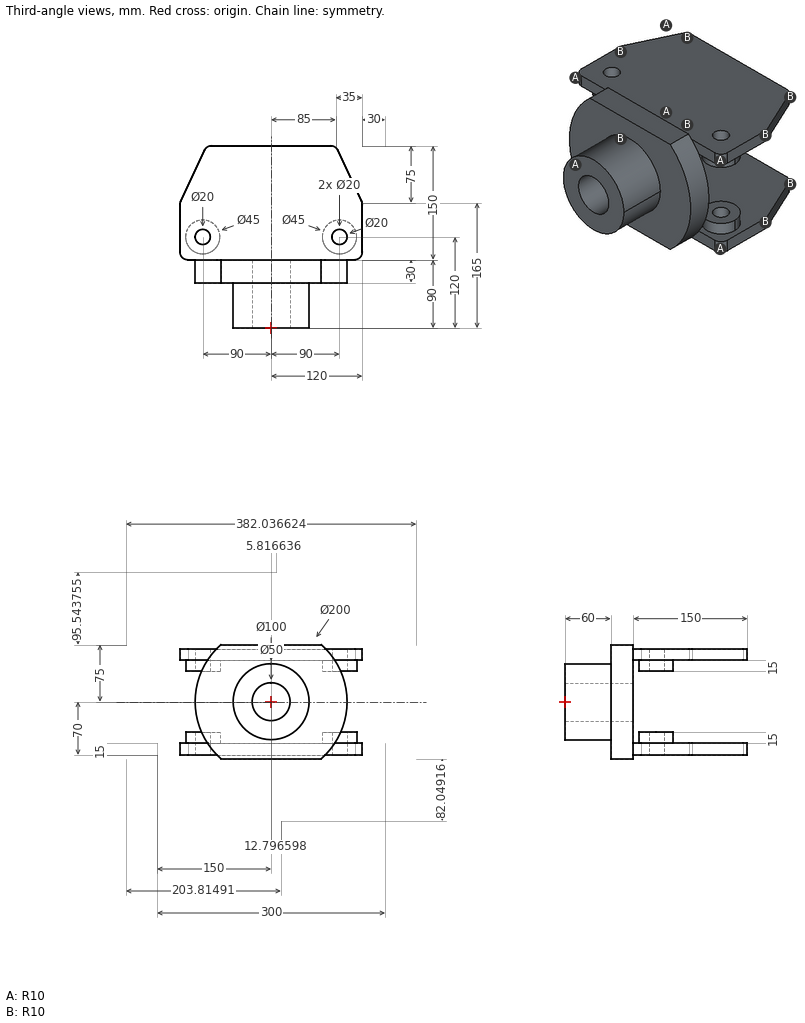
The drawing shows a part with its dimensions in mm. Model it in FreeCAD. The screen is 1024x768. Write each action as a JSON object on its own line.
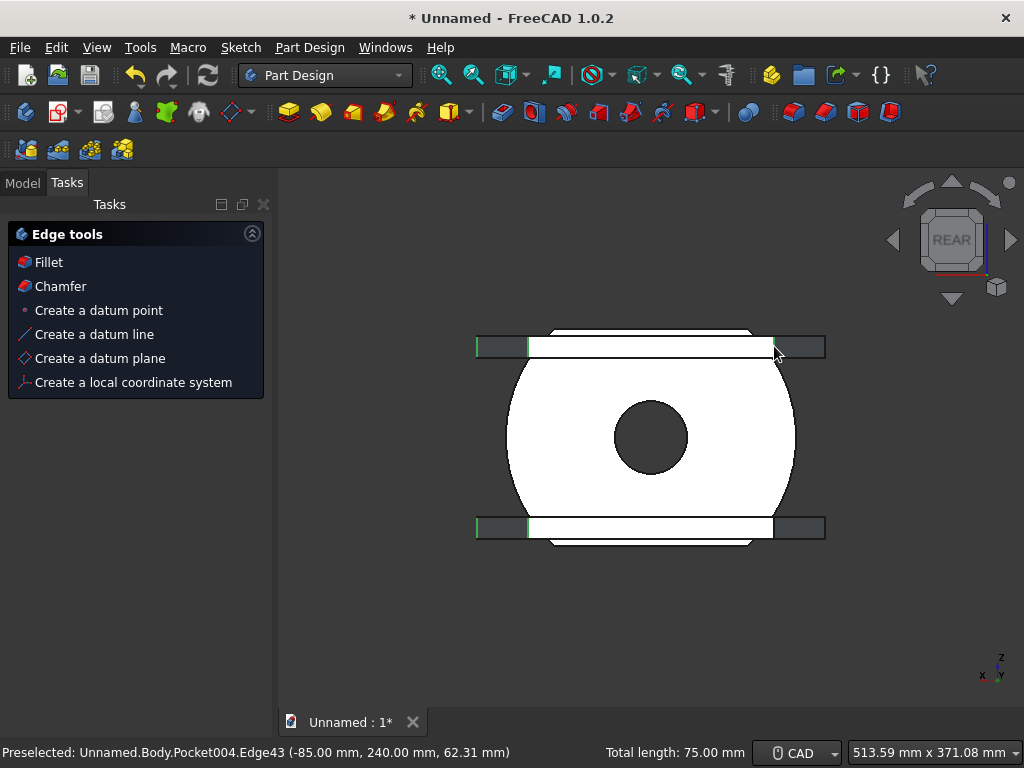
{"action": "left_click", "coordinate": [774, 527], "text": "ctrl"}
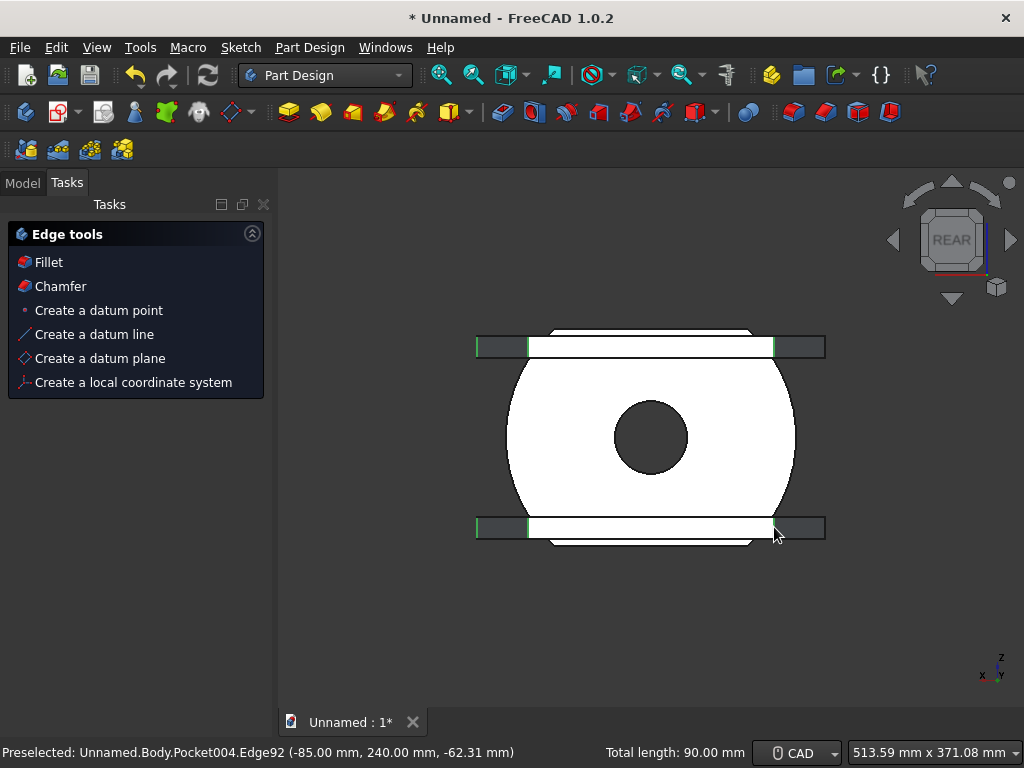
{"action": "scroll", "coordinate": [825, 527], "scroll_direction": "up", "scroll_amount": 4}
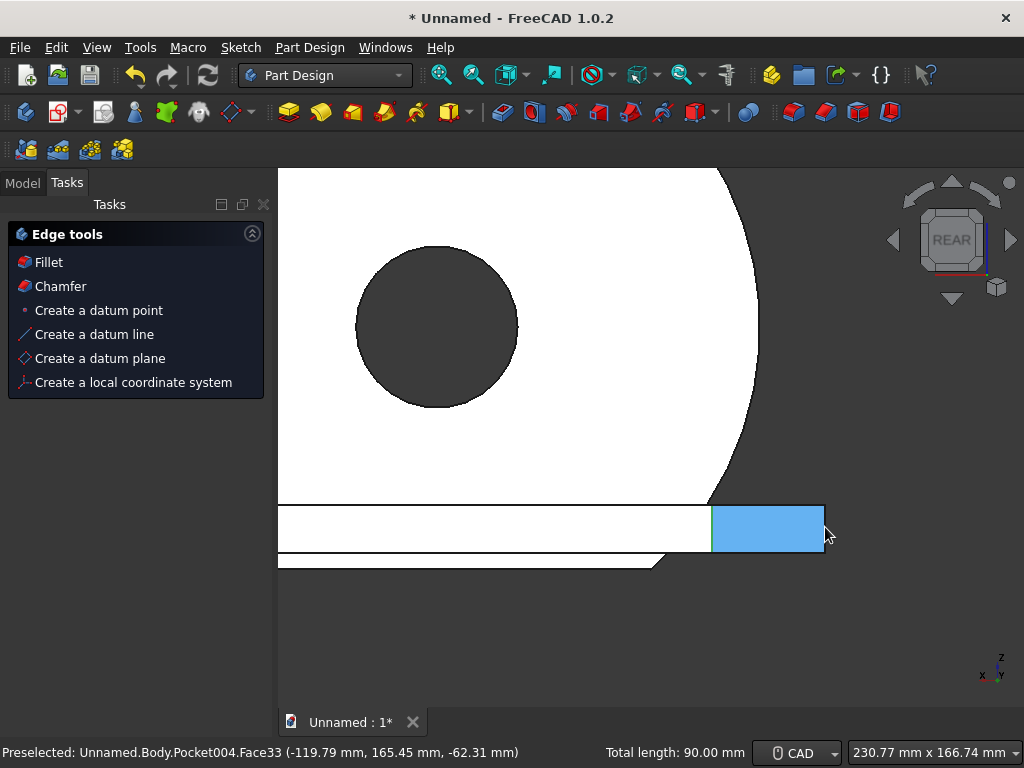
{"action": "left_click", "coordinate": [442, 76]}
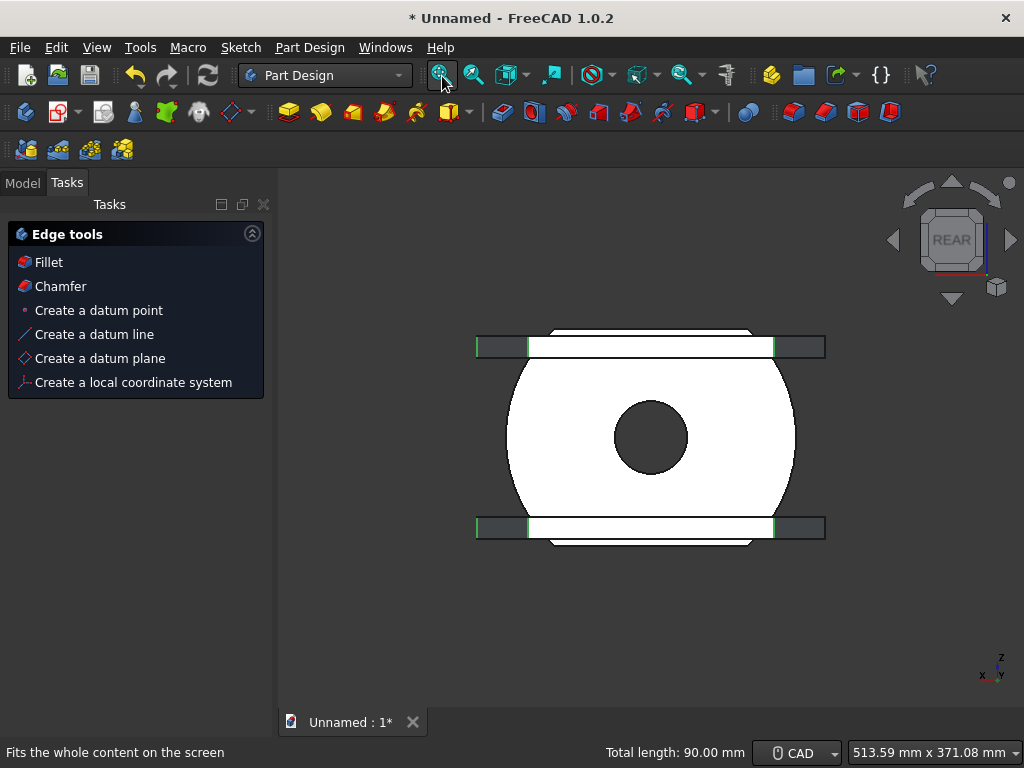
{"action": "key", "text": "6"}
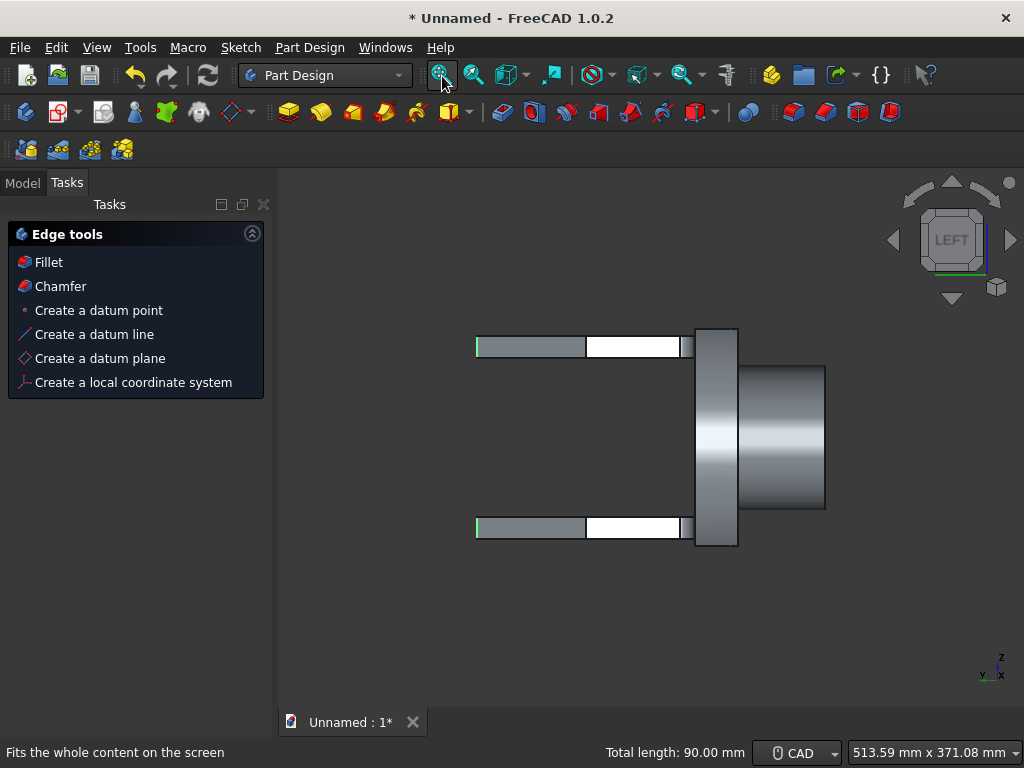
{"action": "left_click", "coordinate": [586, 527], "text": "ctrl"}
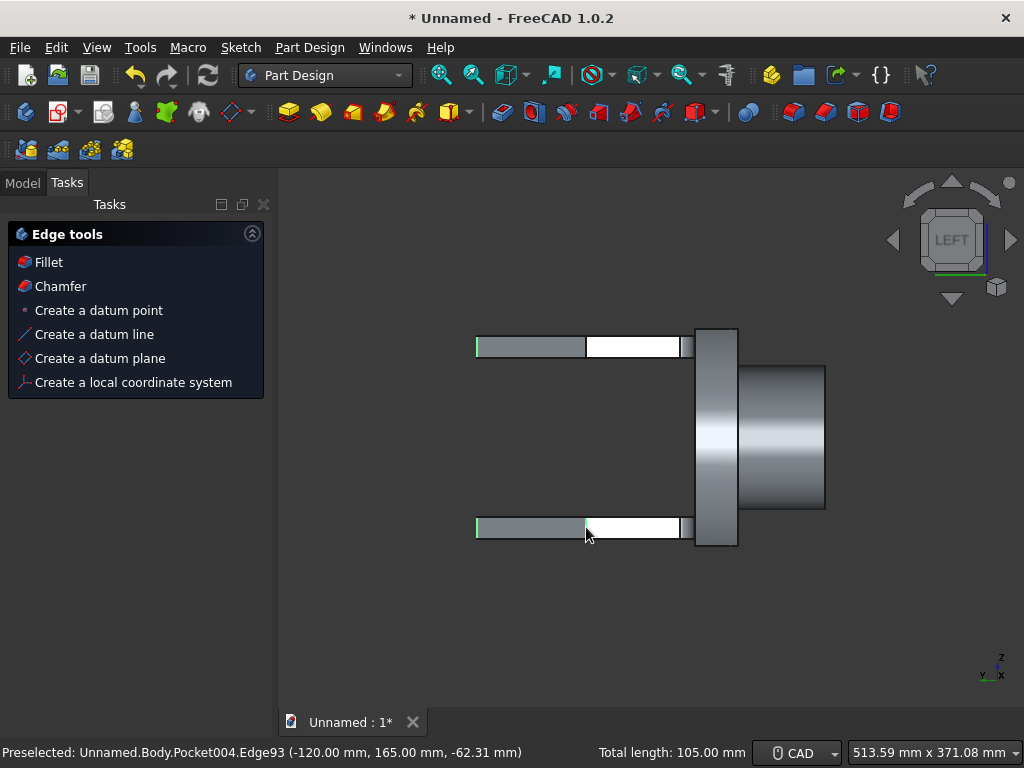
{"action": "left_click", "coordinate": [586, 346], "text": "ctrl"}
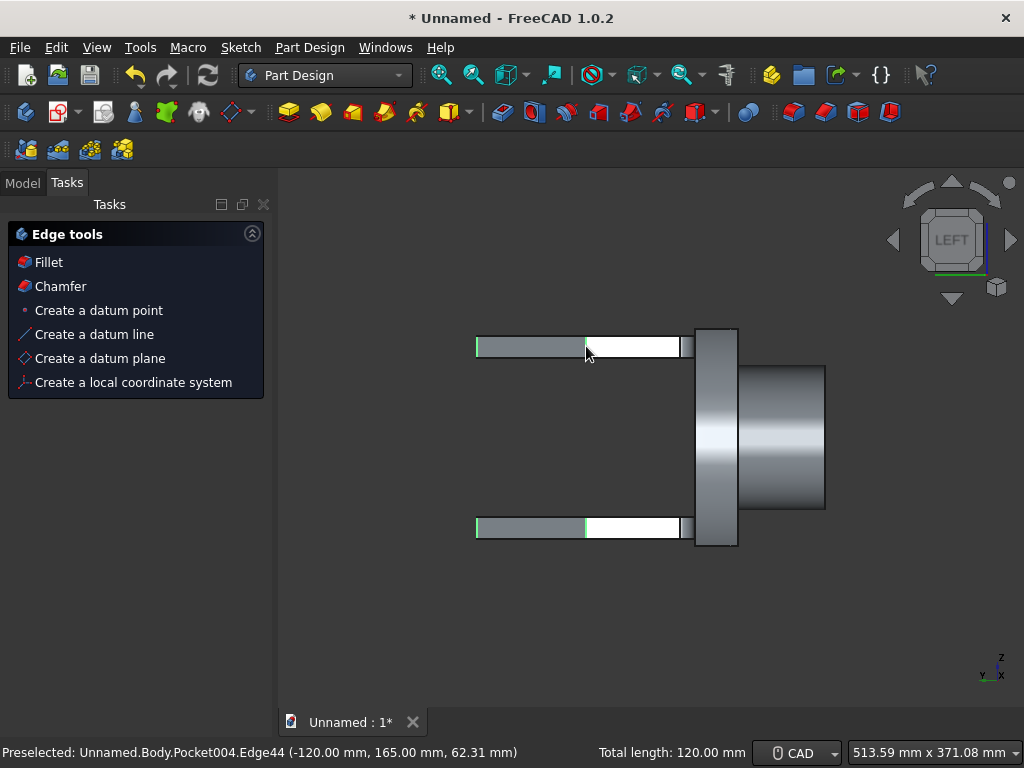
{"action": "left_click", "coordinate": [794, 112]}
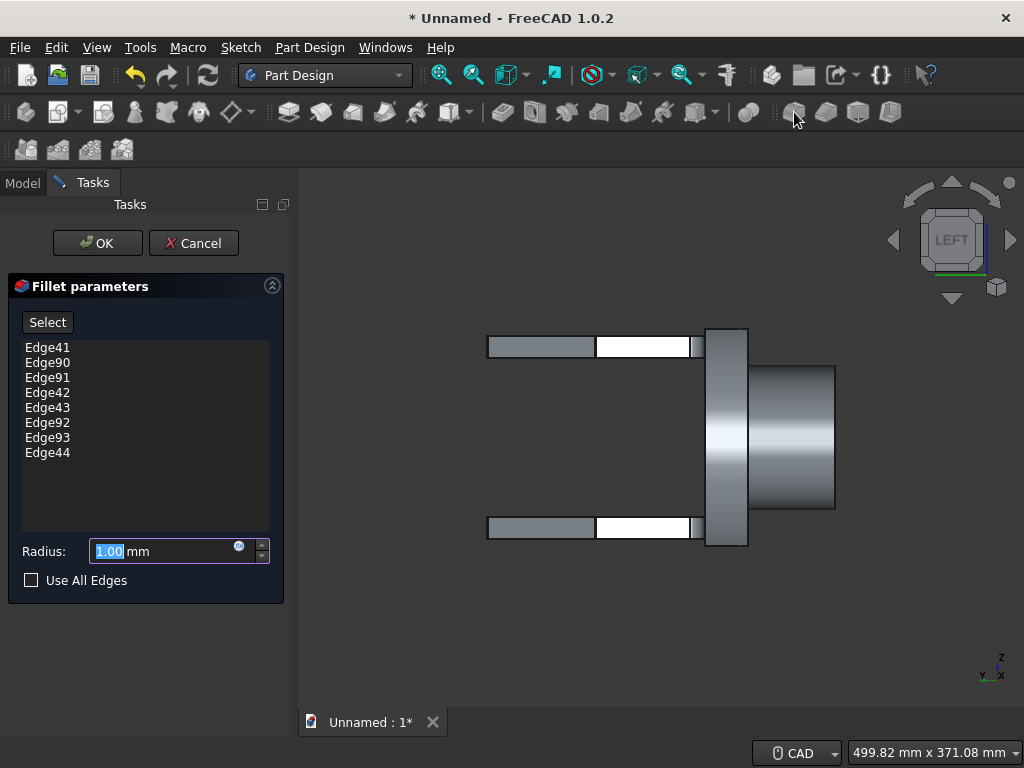
{"action": "type", "text": "10"}
{"action": "key", "text": "Tab"}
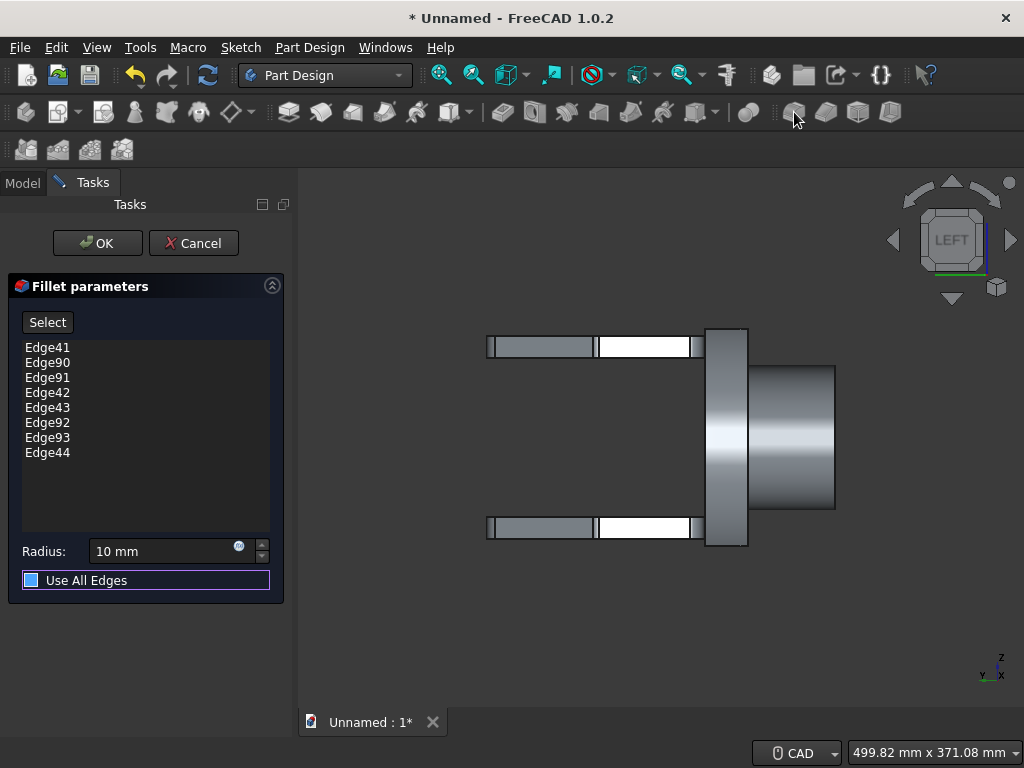
{"action": "left_click", "coordinate": [98, 243]}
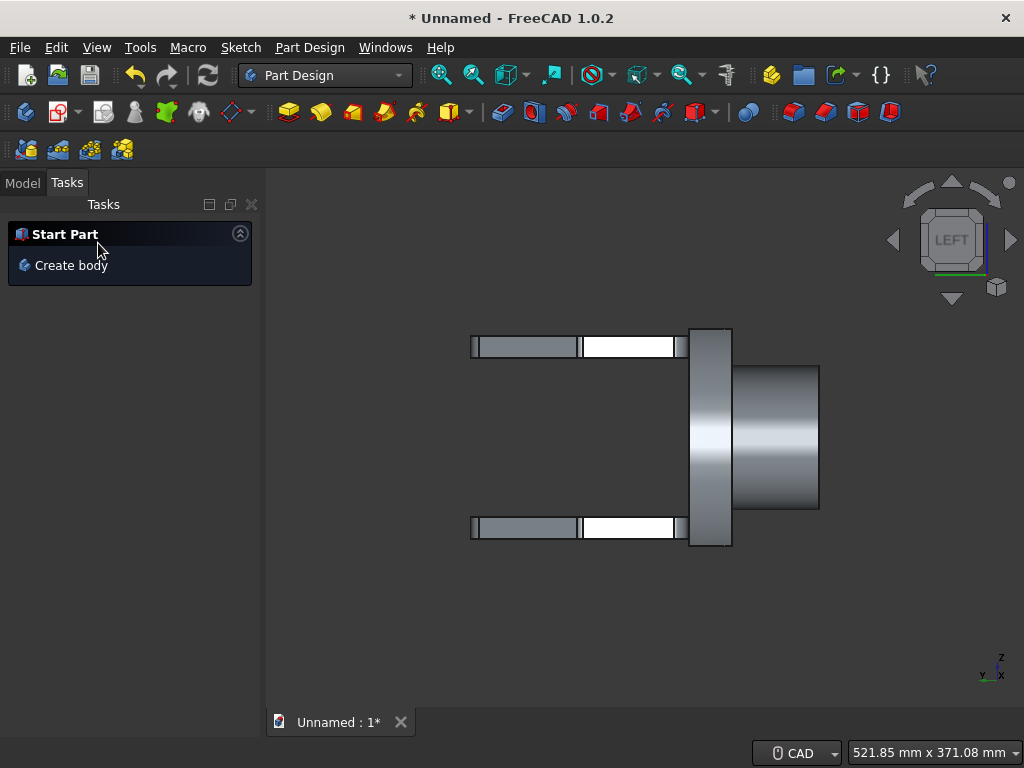
{"action": "left_click", "coordinate": [26, 112]}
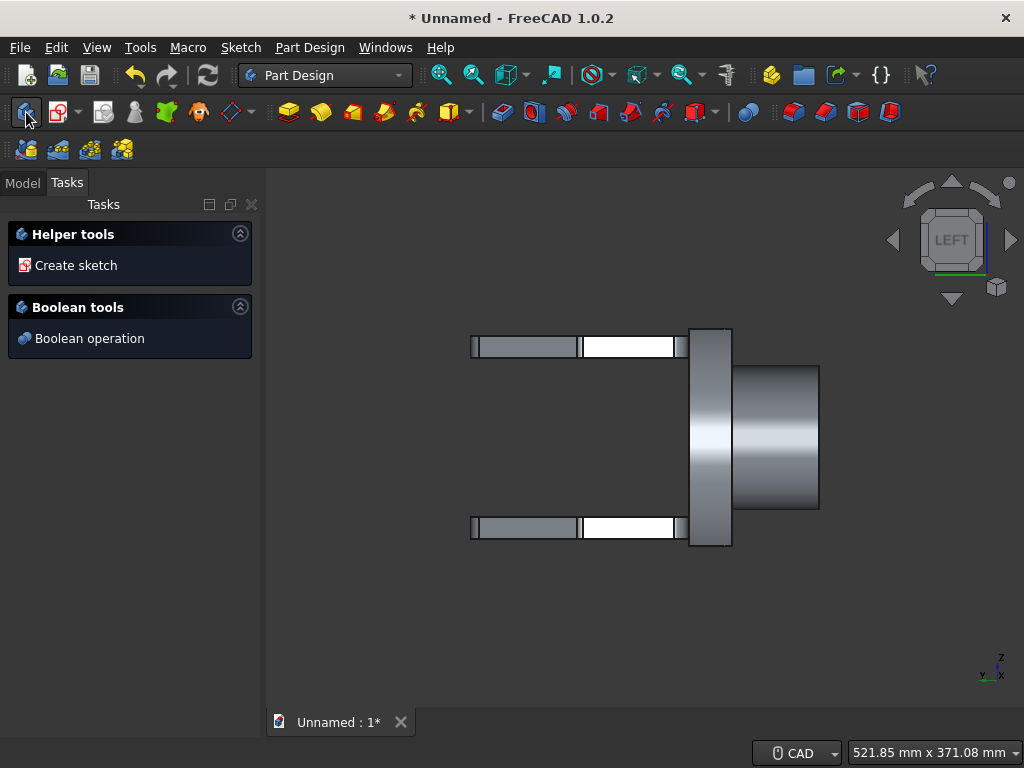
{"action": "left_click", "coordinate": [23, 182]}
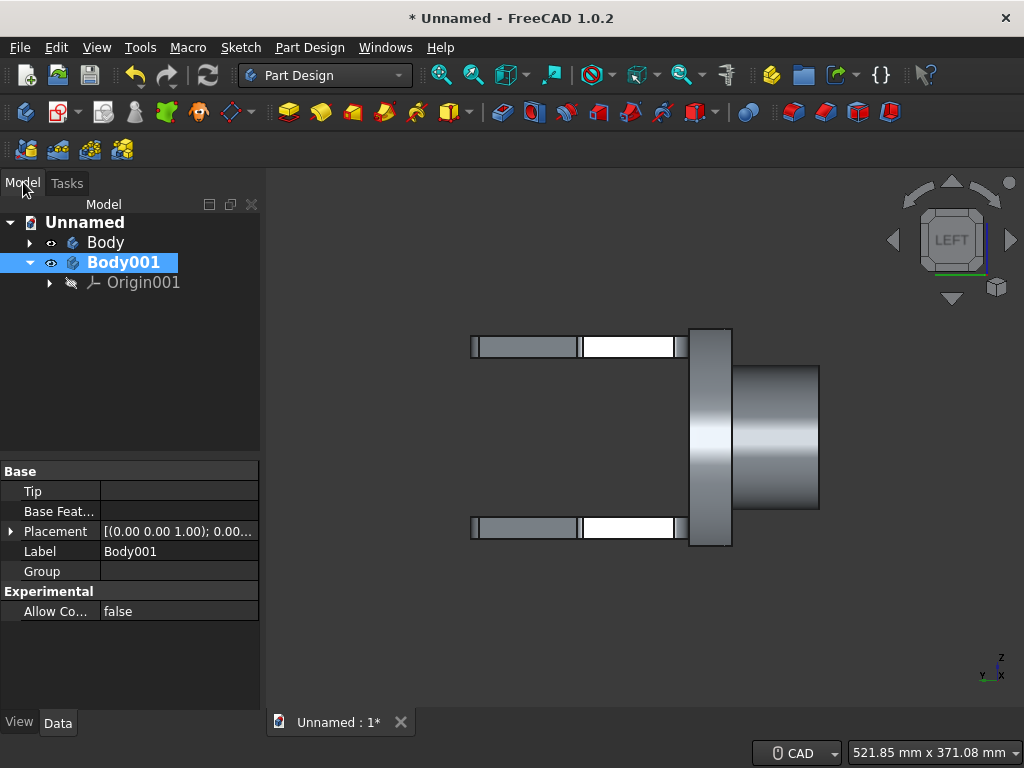
{"action": "left_click", "coordinate": [50, 283]}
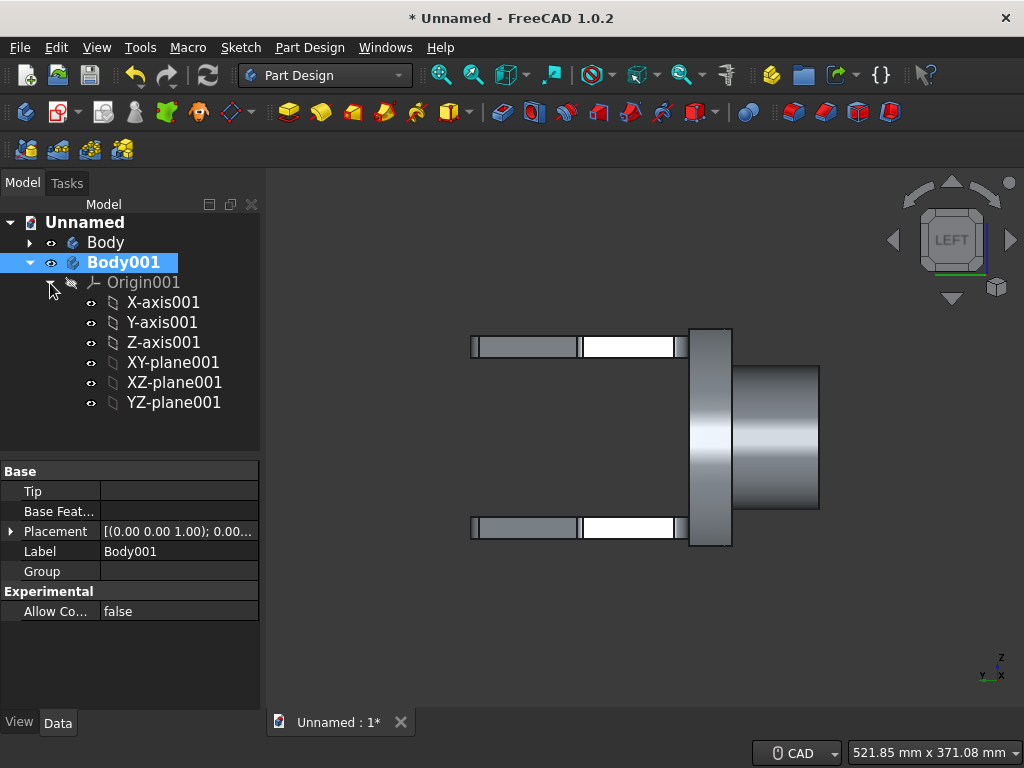
{"action": "left_click", "coordinate": [136, 363]}